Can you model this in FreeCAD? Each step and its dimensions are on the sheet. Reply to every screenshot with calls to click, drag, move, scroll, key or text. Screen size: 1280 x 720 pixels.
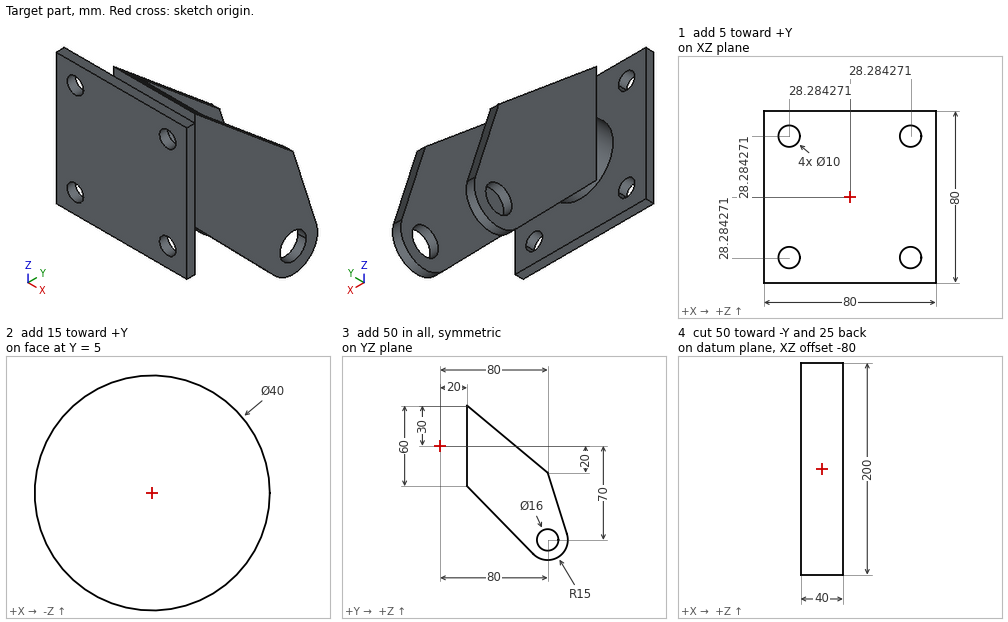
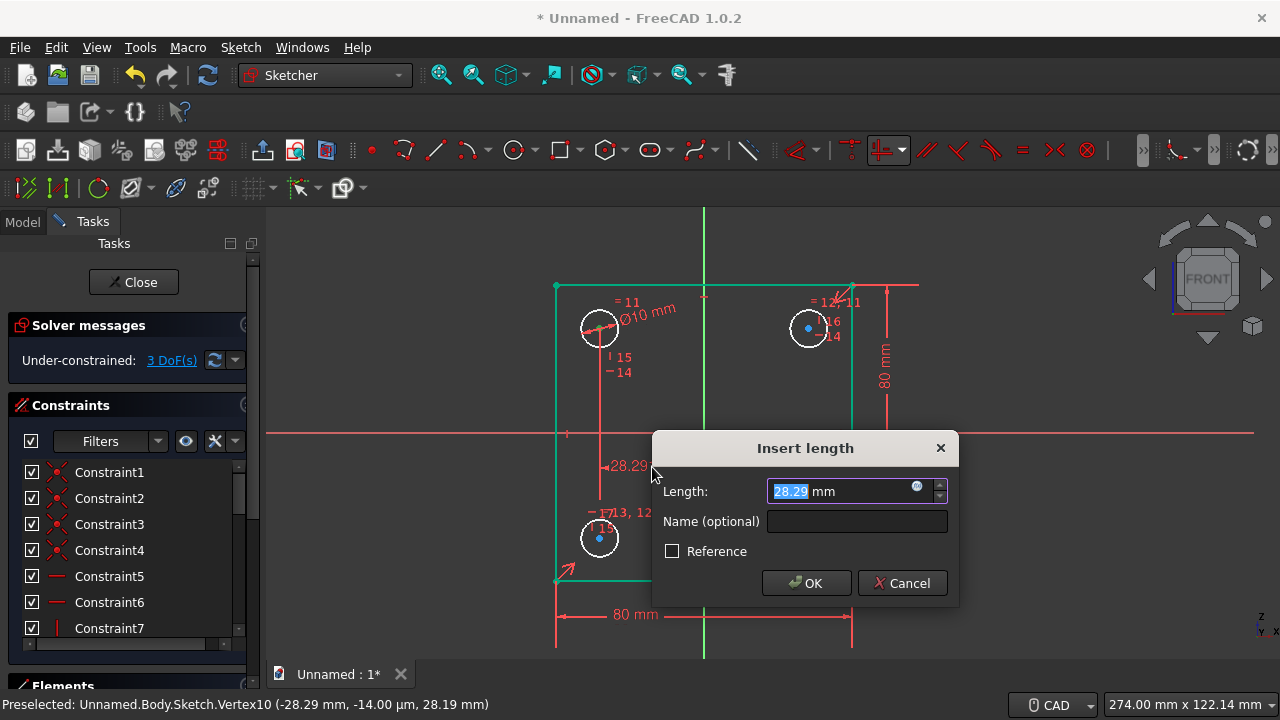
text(28.284271)
key(Return)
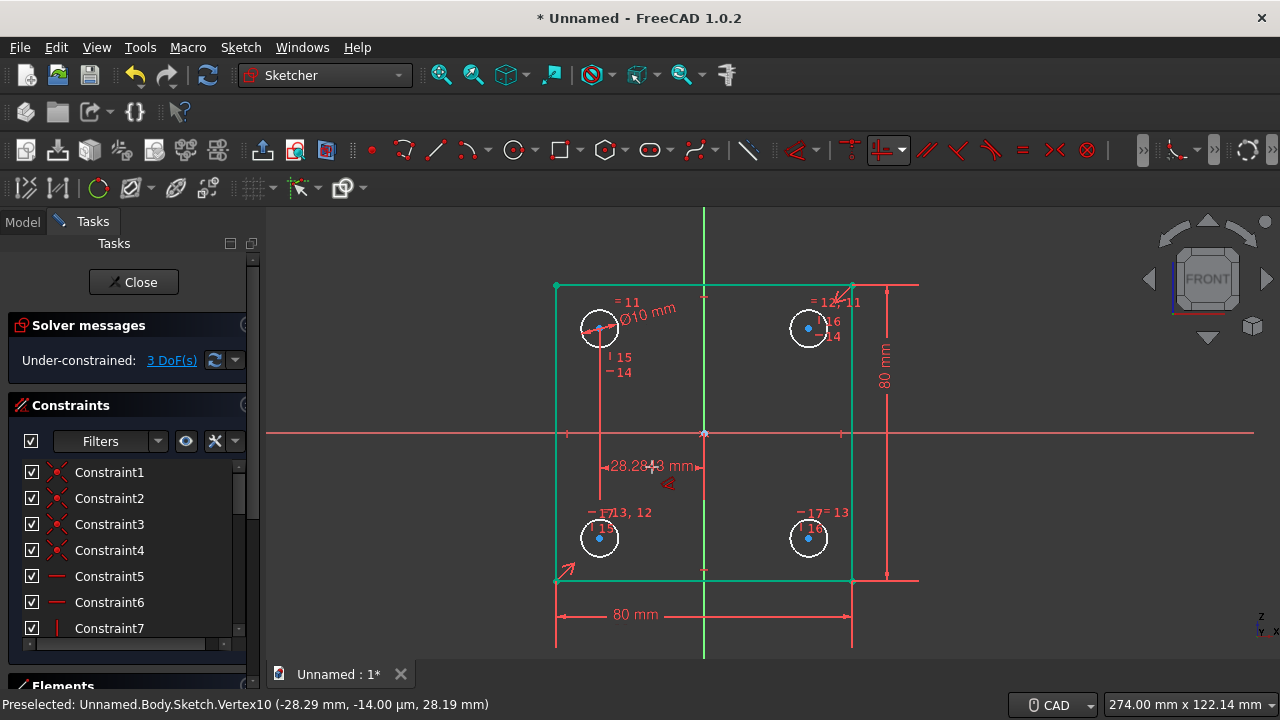
click(600, 329)
click(738, 381)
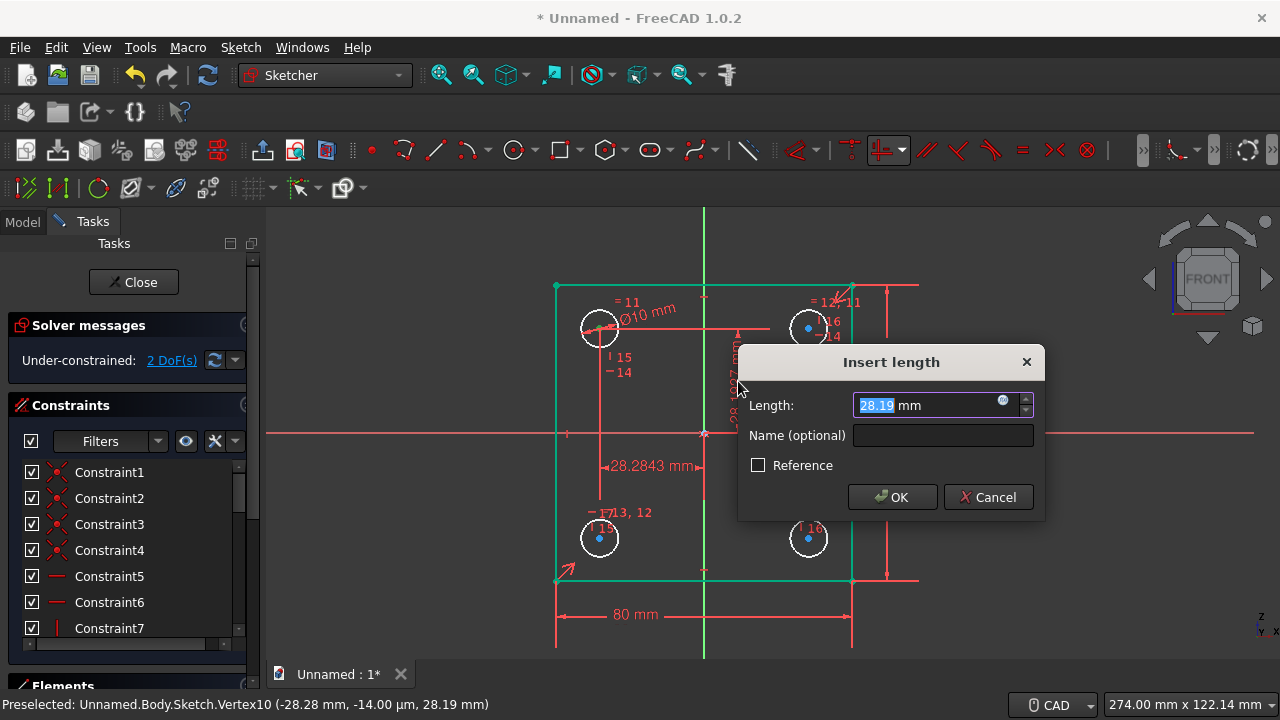
text(28.284271)
key(Return)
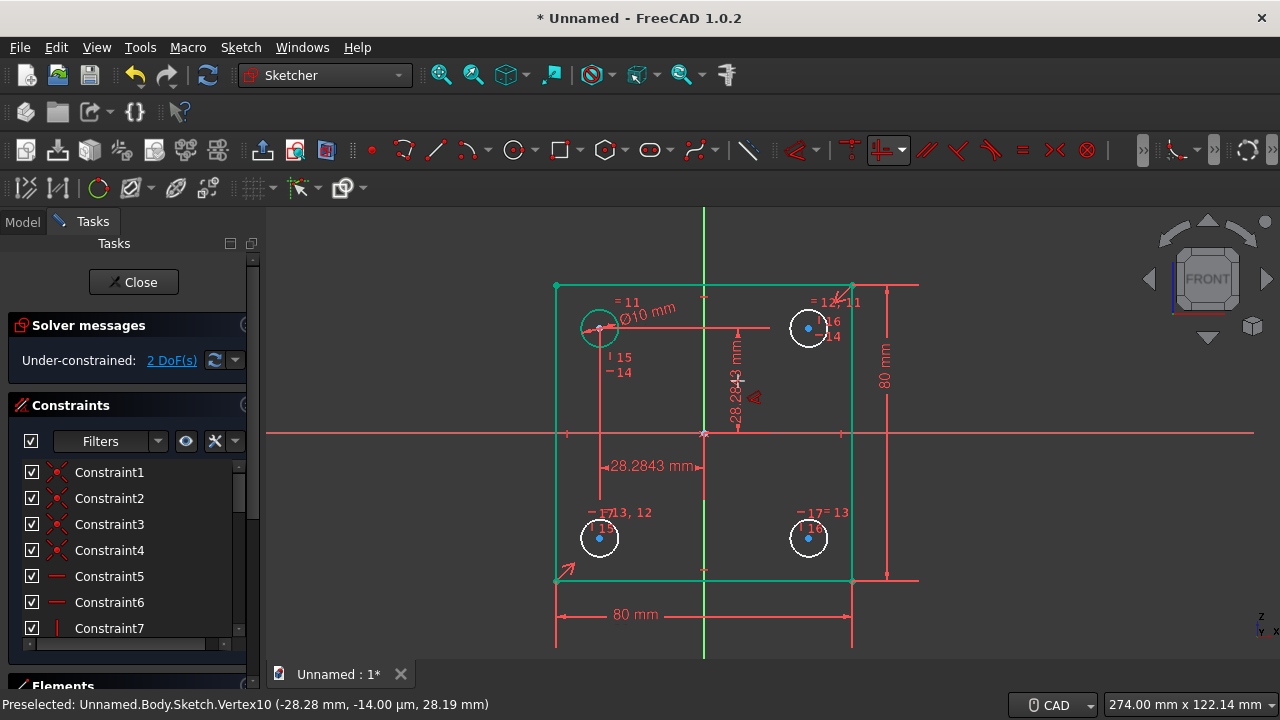
click(809, 328)
click(757, 467)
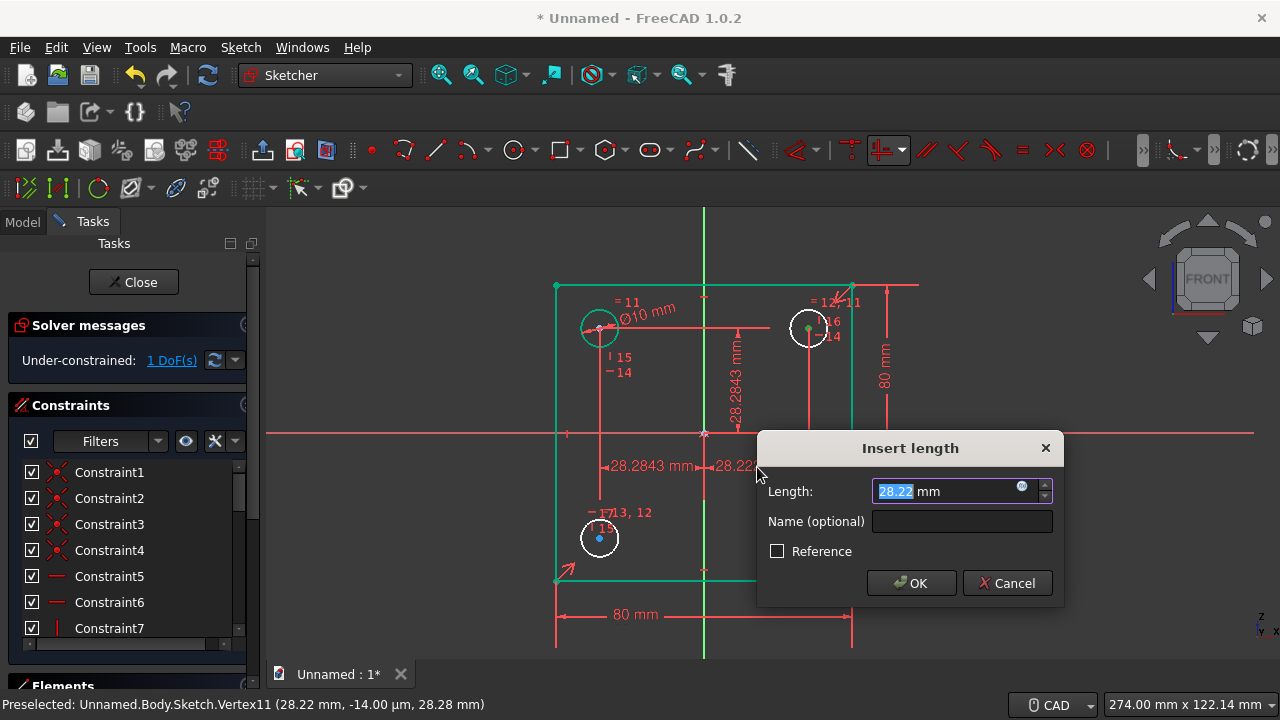
text(28.284271)
key(Return)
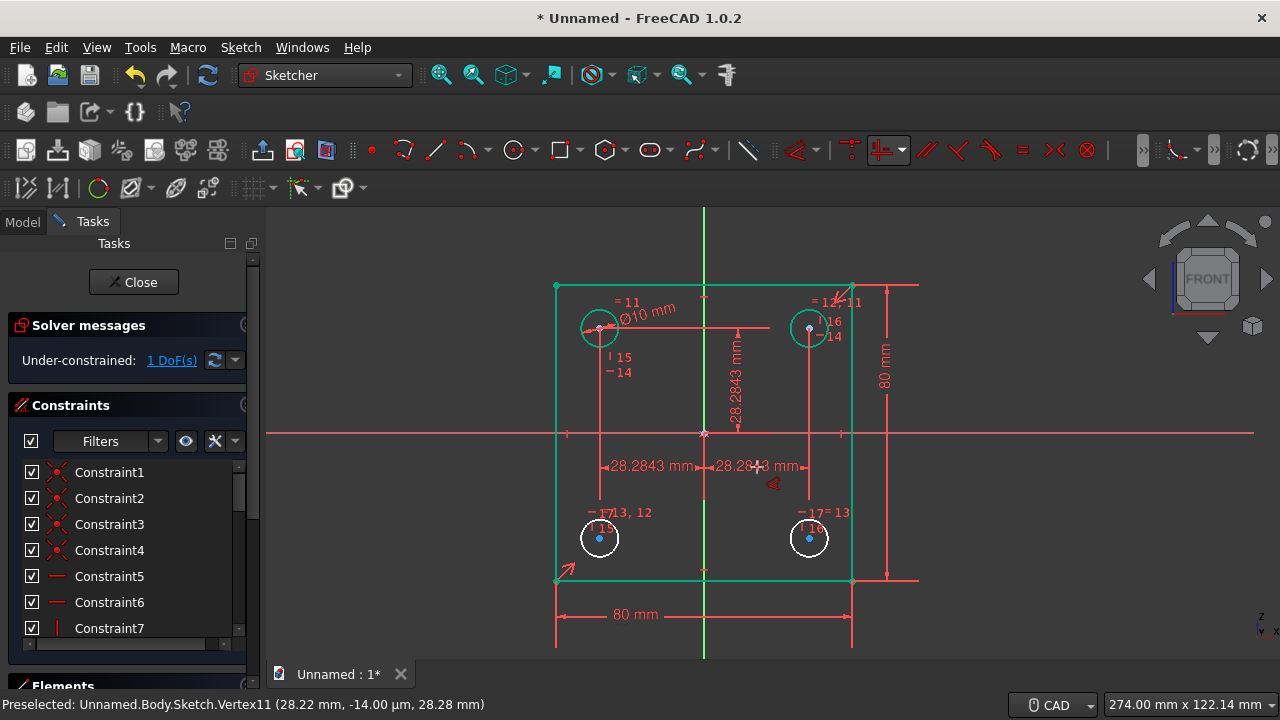
click(600, 538)
click(738, 510)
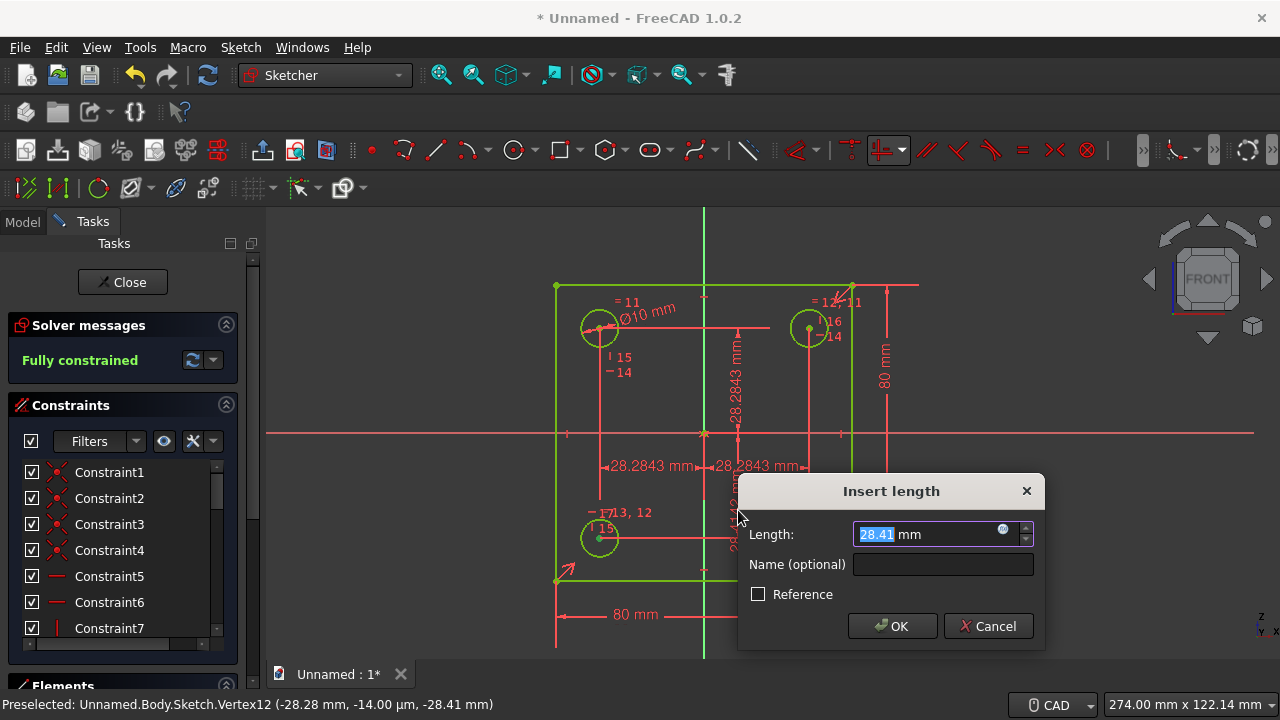
text(28.284271)
key(Return)
key(Escape)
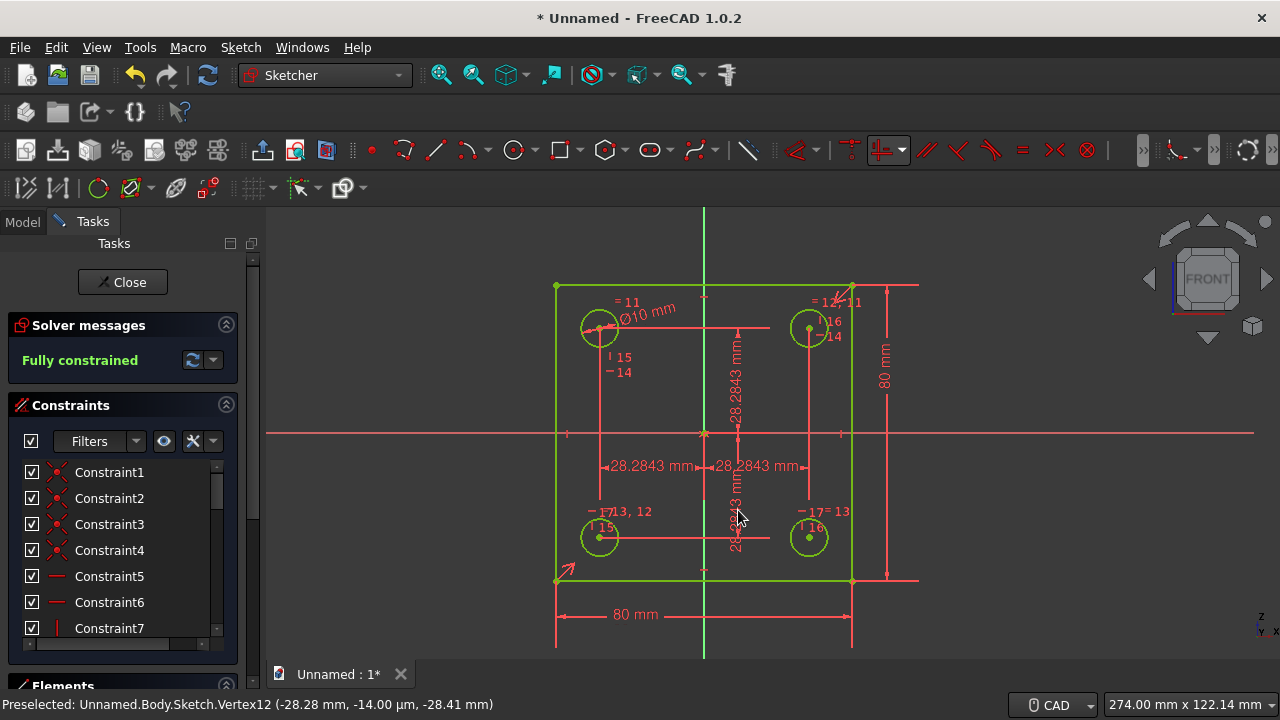
click(123, 282)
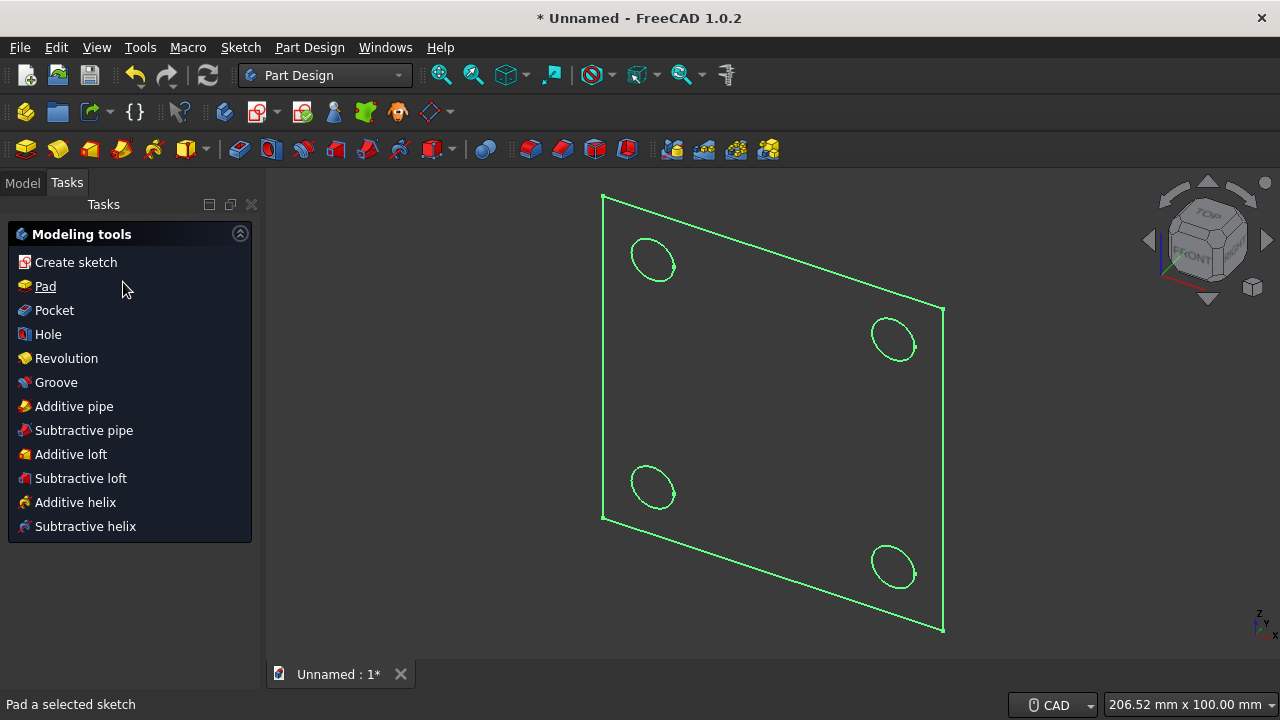
click(26, 150)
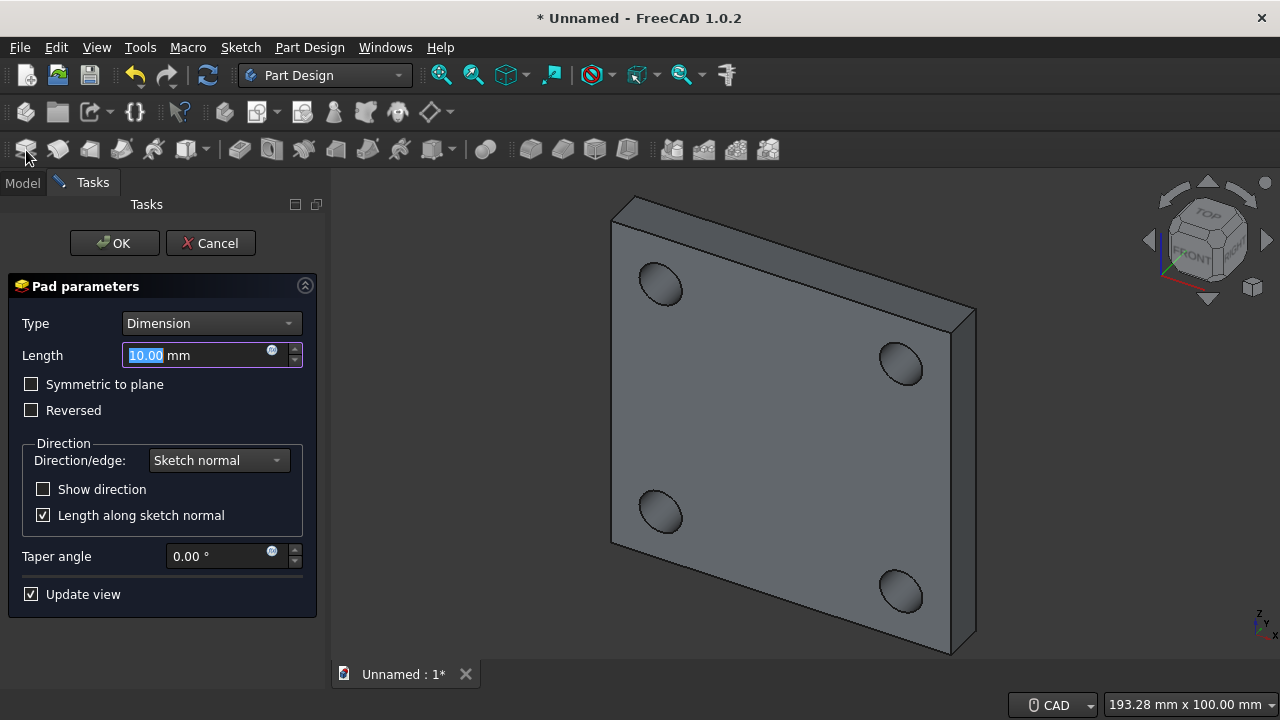
text(5)
key(Tab)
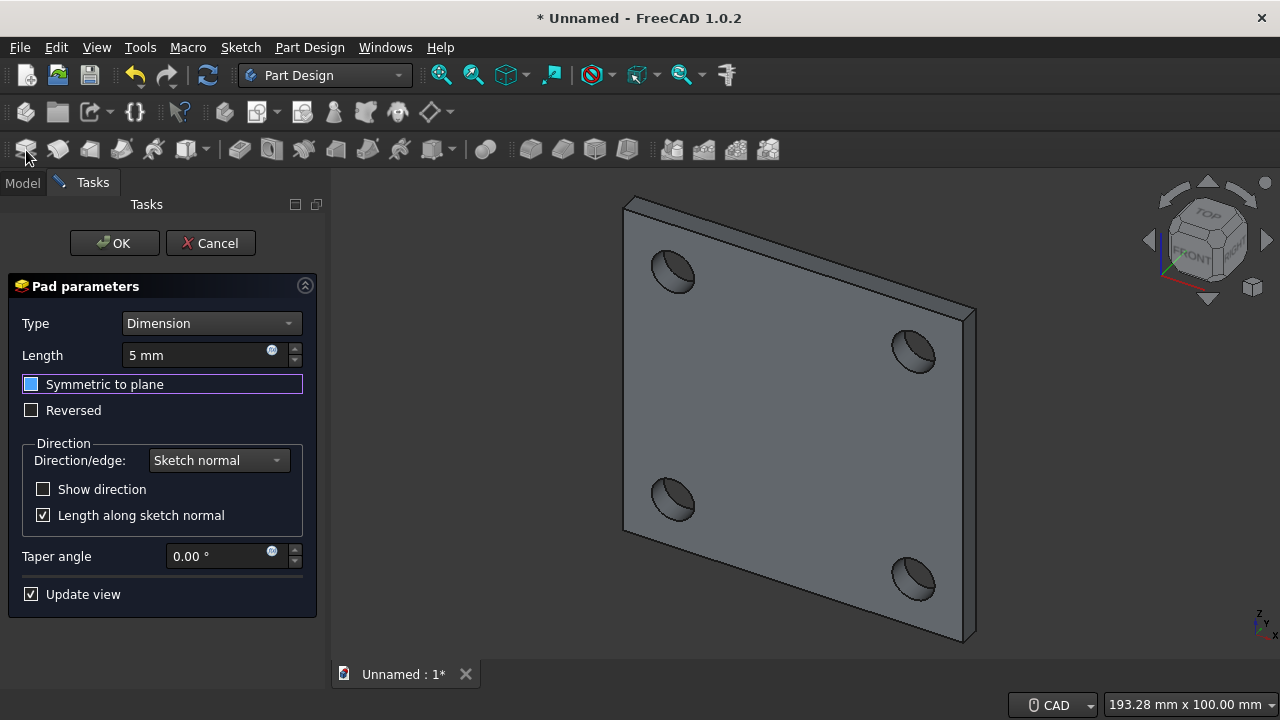
click(30, 410)